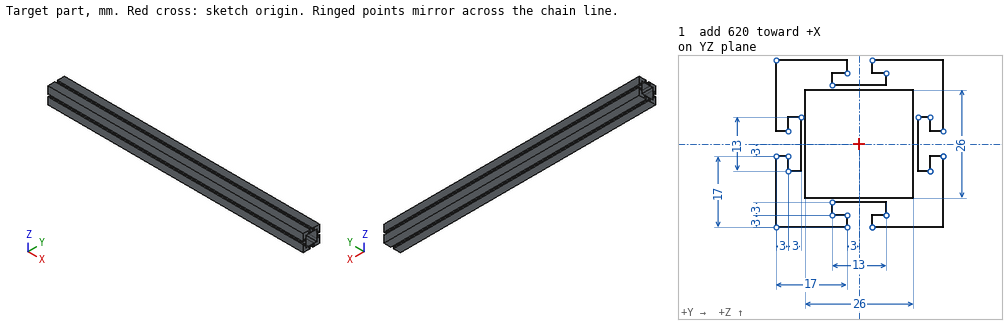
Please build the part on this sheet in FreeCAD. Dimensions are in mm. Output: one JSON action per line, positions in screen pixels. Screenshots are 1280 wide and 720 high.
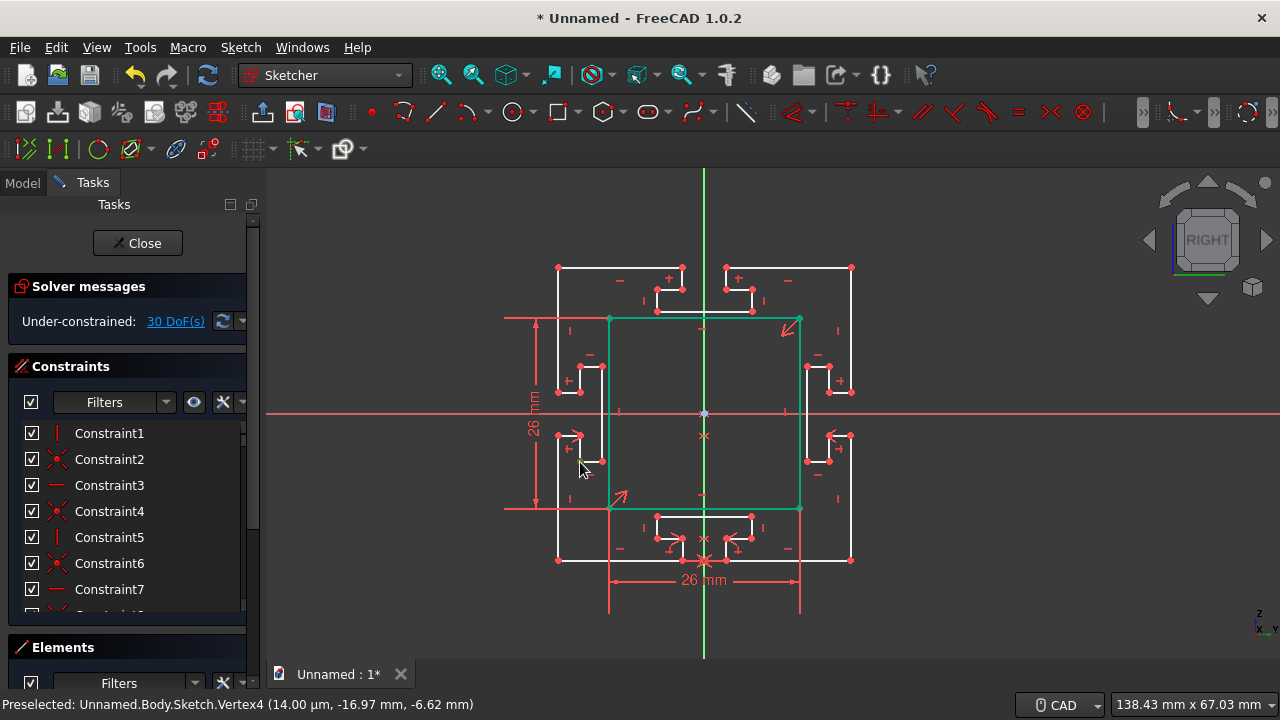
{"action": "left_click", "coordinate": [829, 462]}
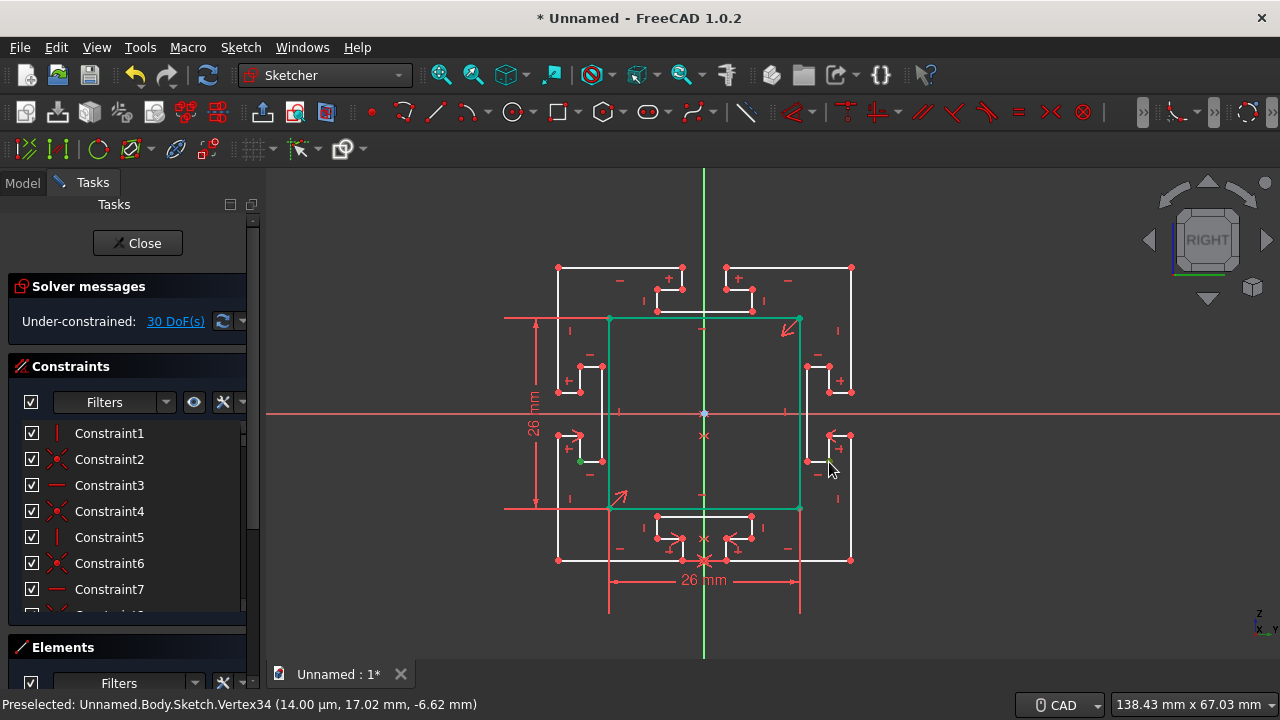
{"action": "left_click", "coordinate": [704, 600]}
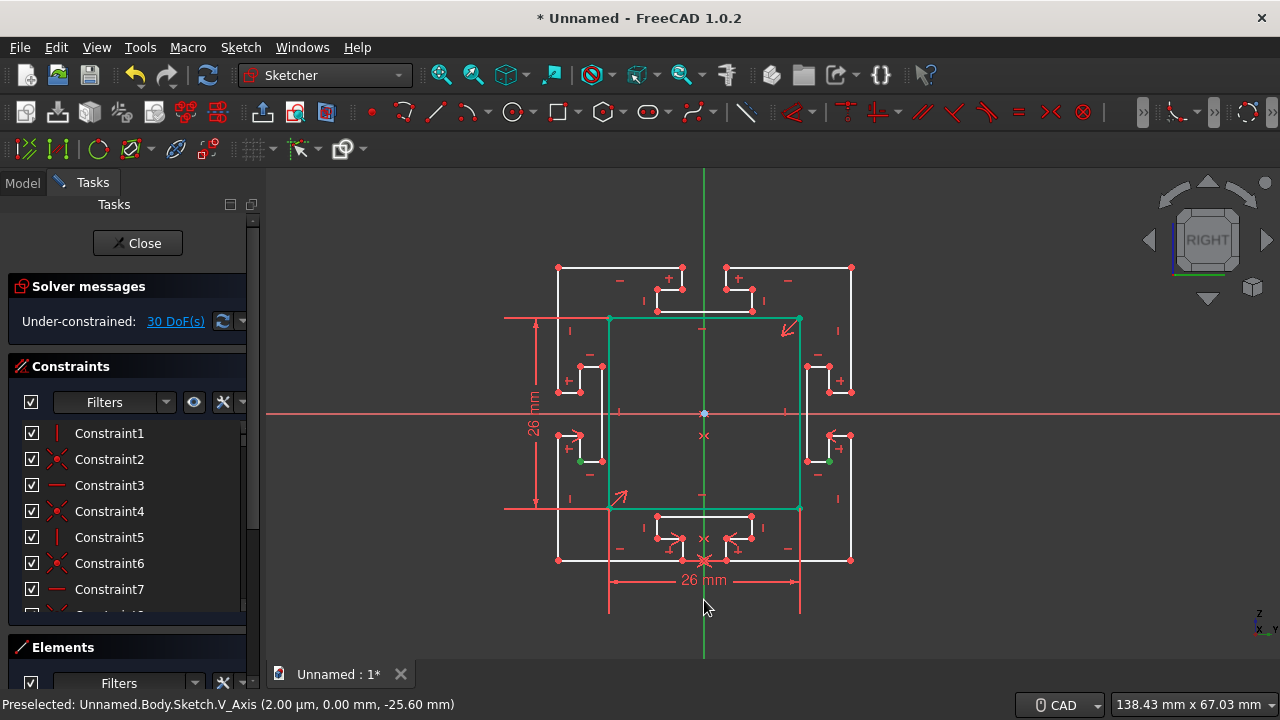
{"action": "key", "text": "s"}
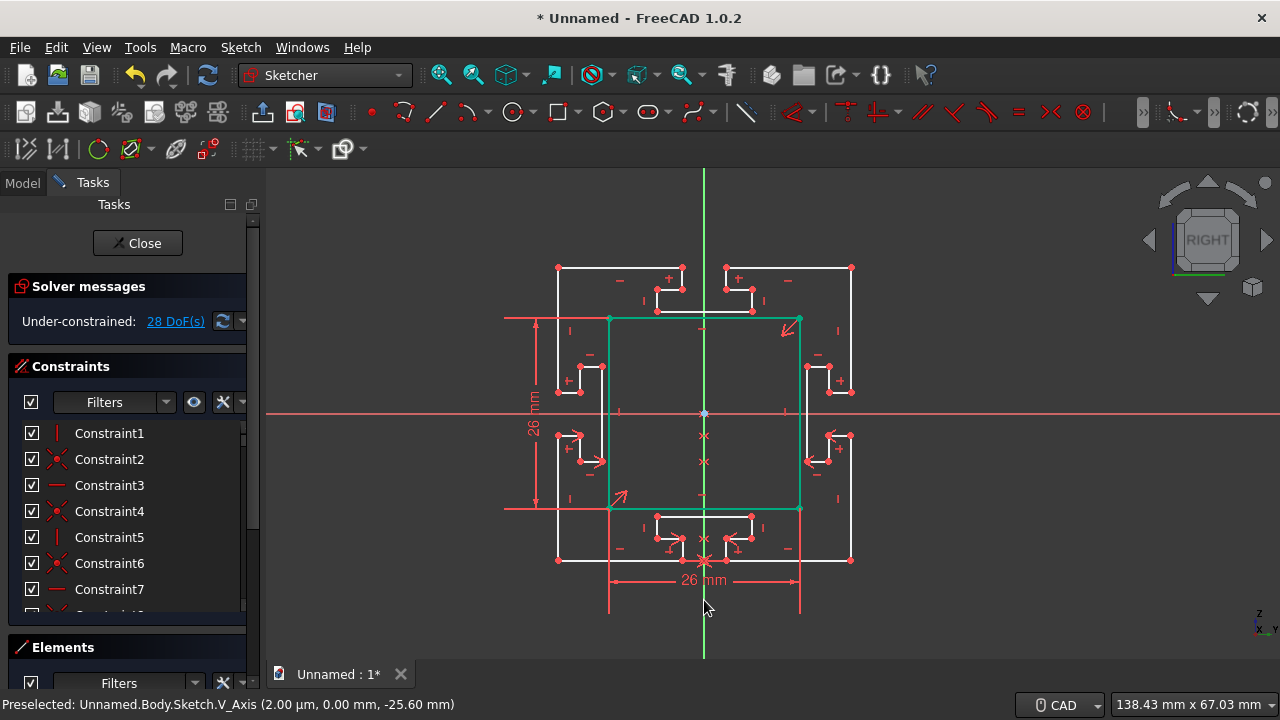
{"action": "left_click", "coordinate": [602, 367]}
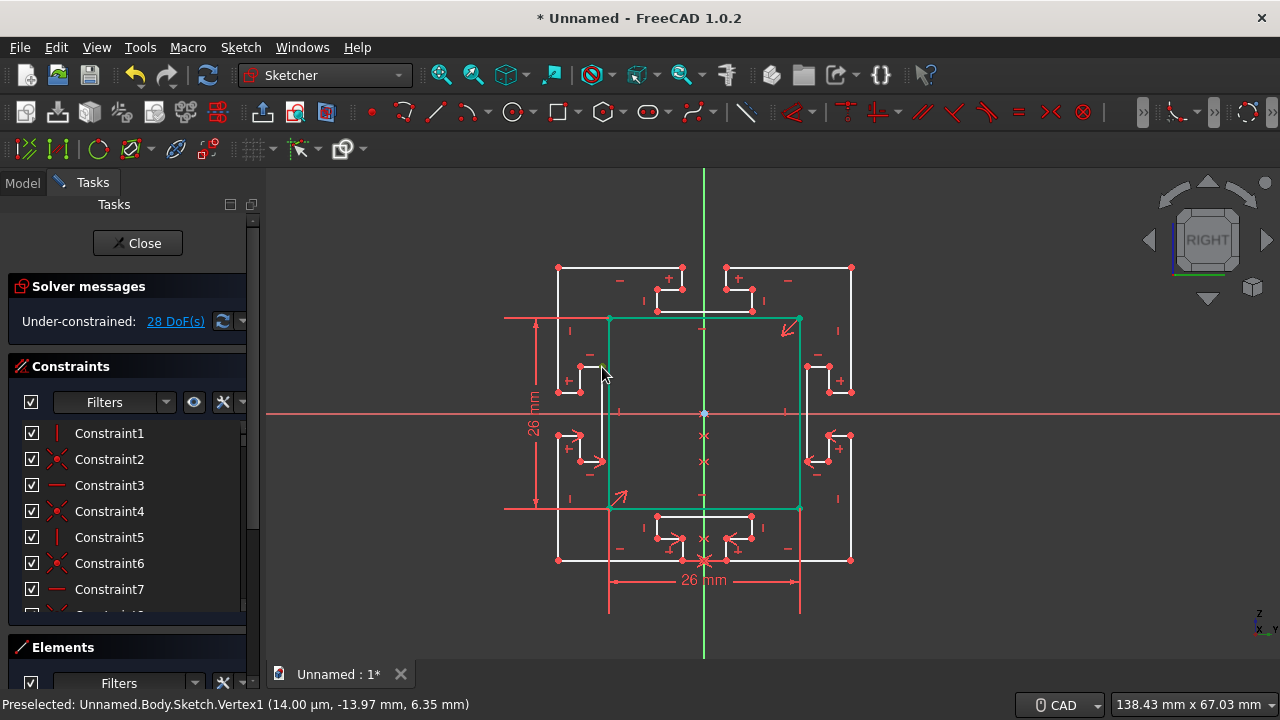
{"action": "left_click", "coordinate": [807, 367]}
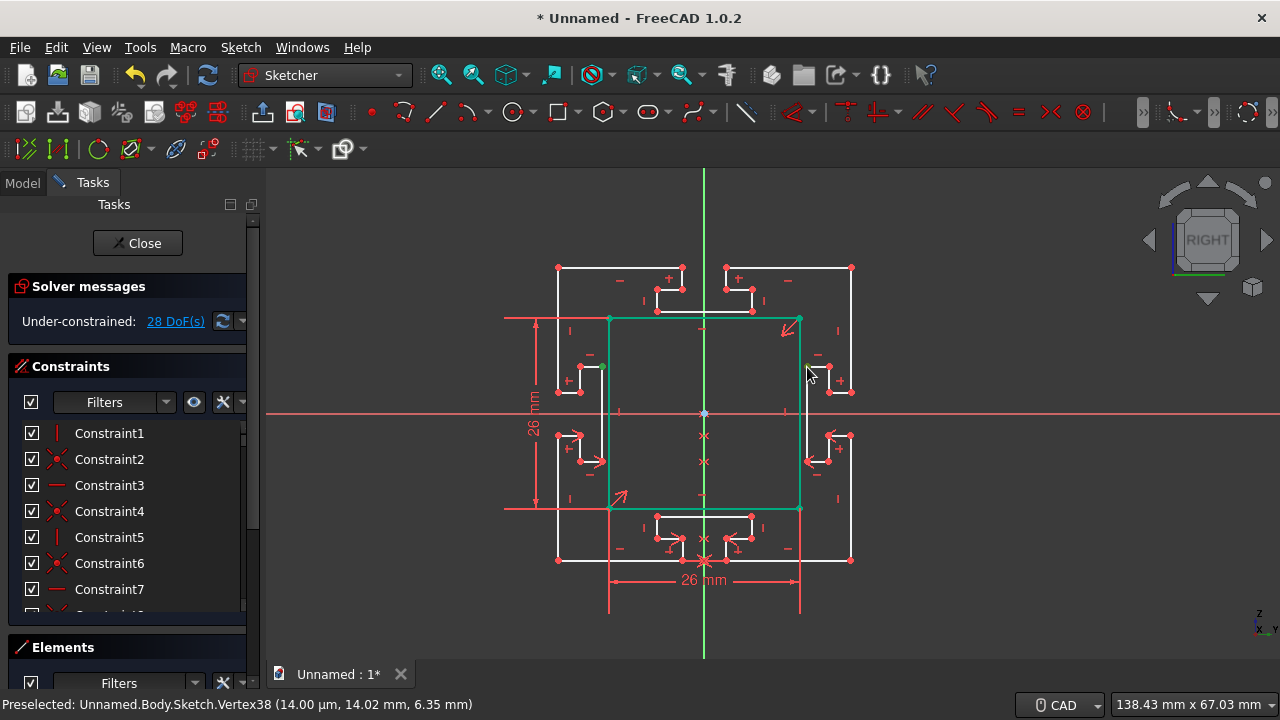
{"action": "left_click", "coordinate": [704, 600]}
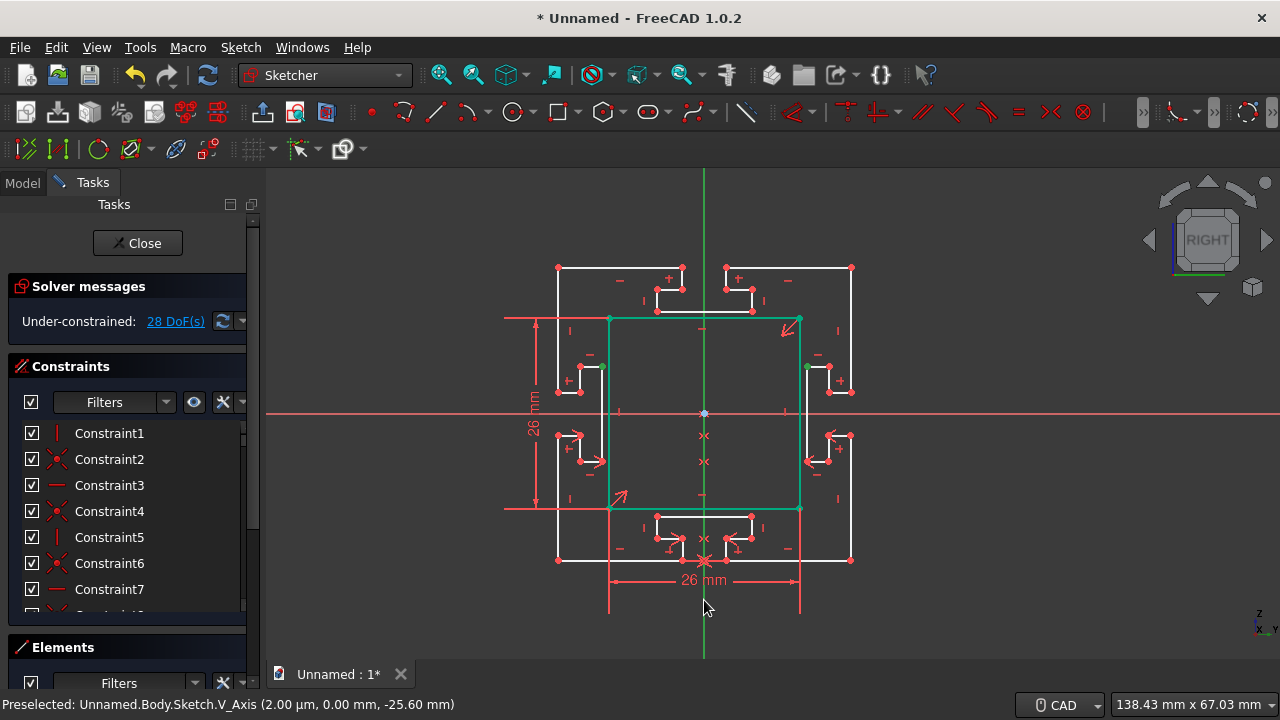
{"action": "key", "text": "s"}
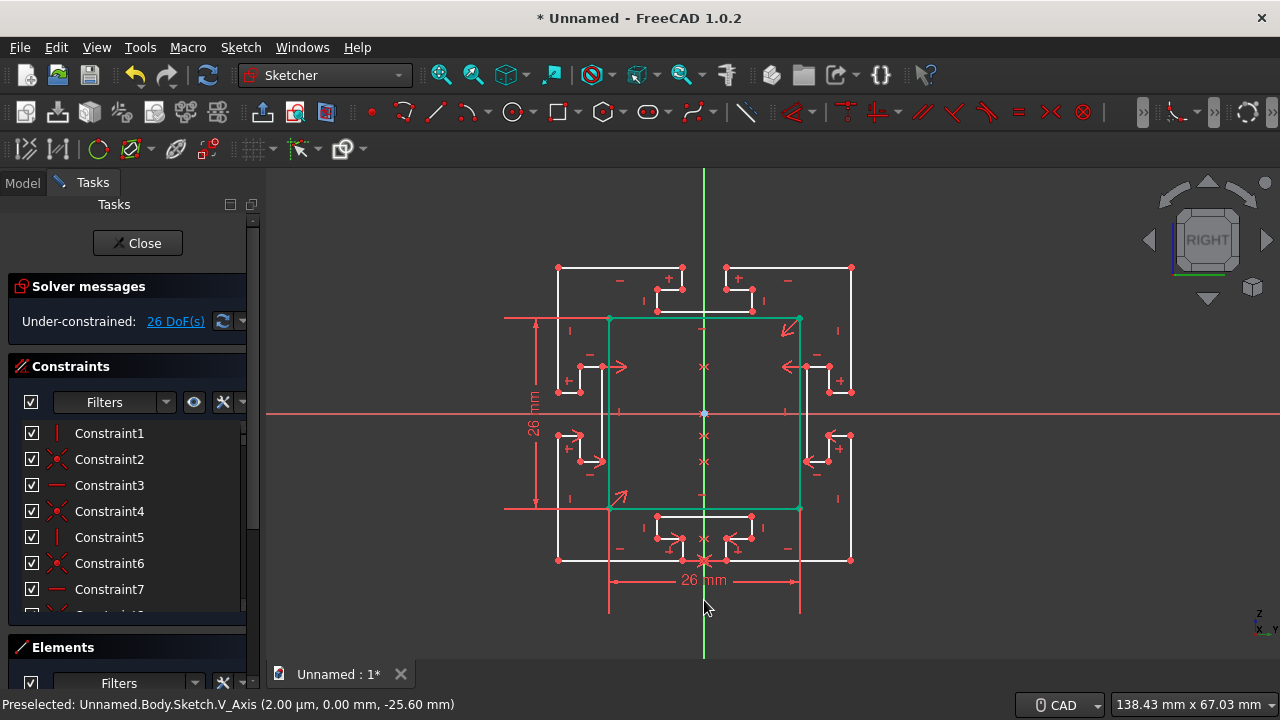
{"action": "left_click", "coordinate": [829, 462]}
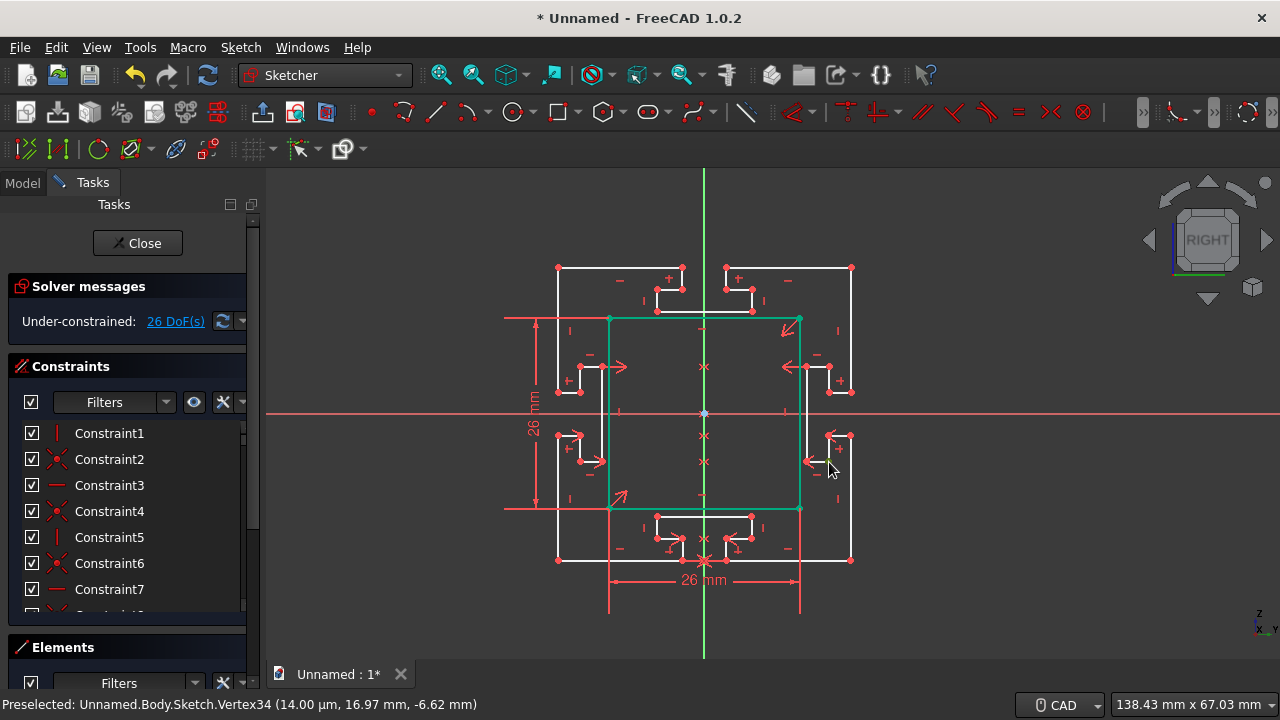
{"action": "left_click", "coordinate": [829, 367]}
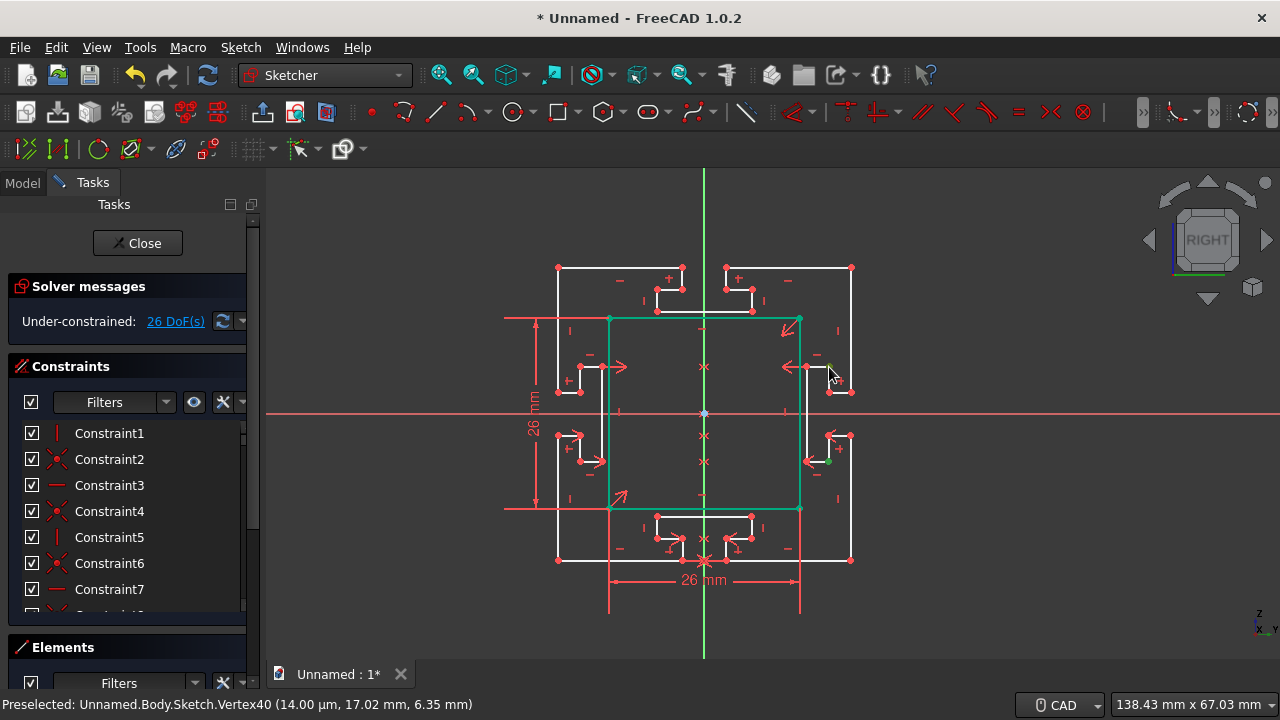
{"action": "left_click", "coordinate": [353, 414]}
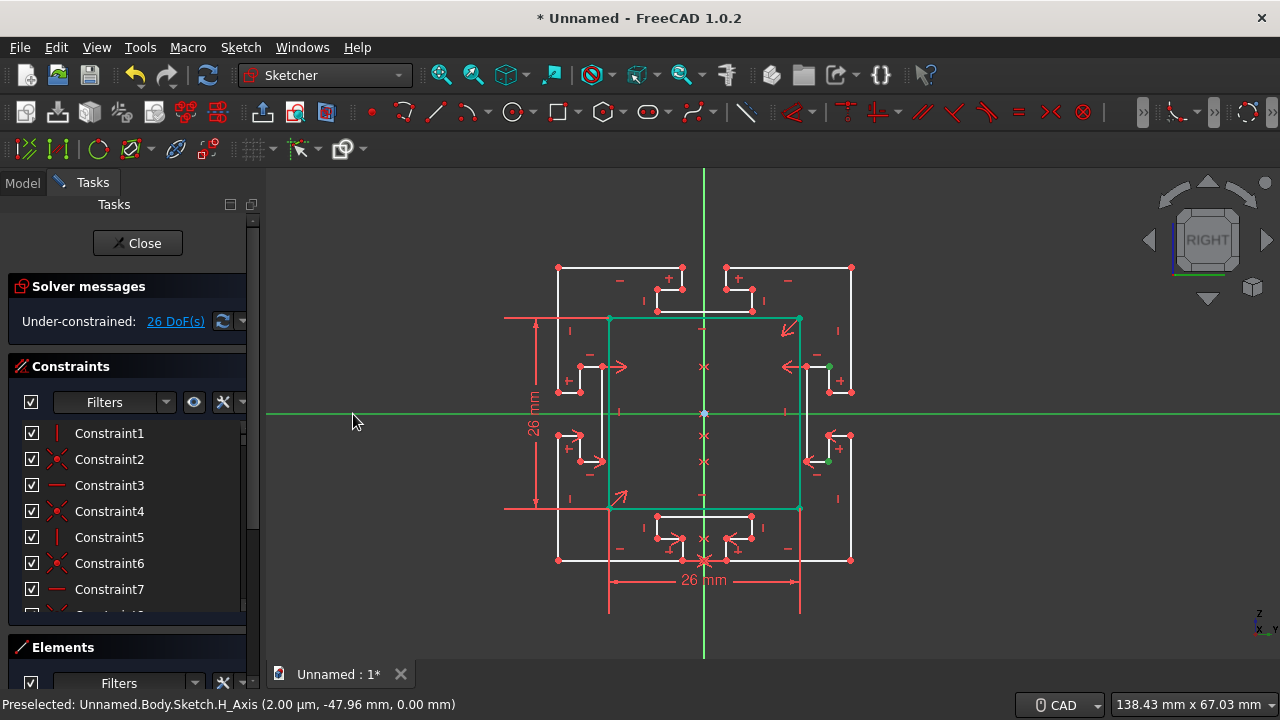
{"action": "key", "text": "s"}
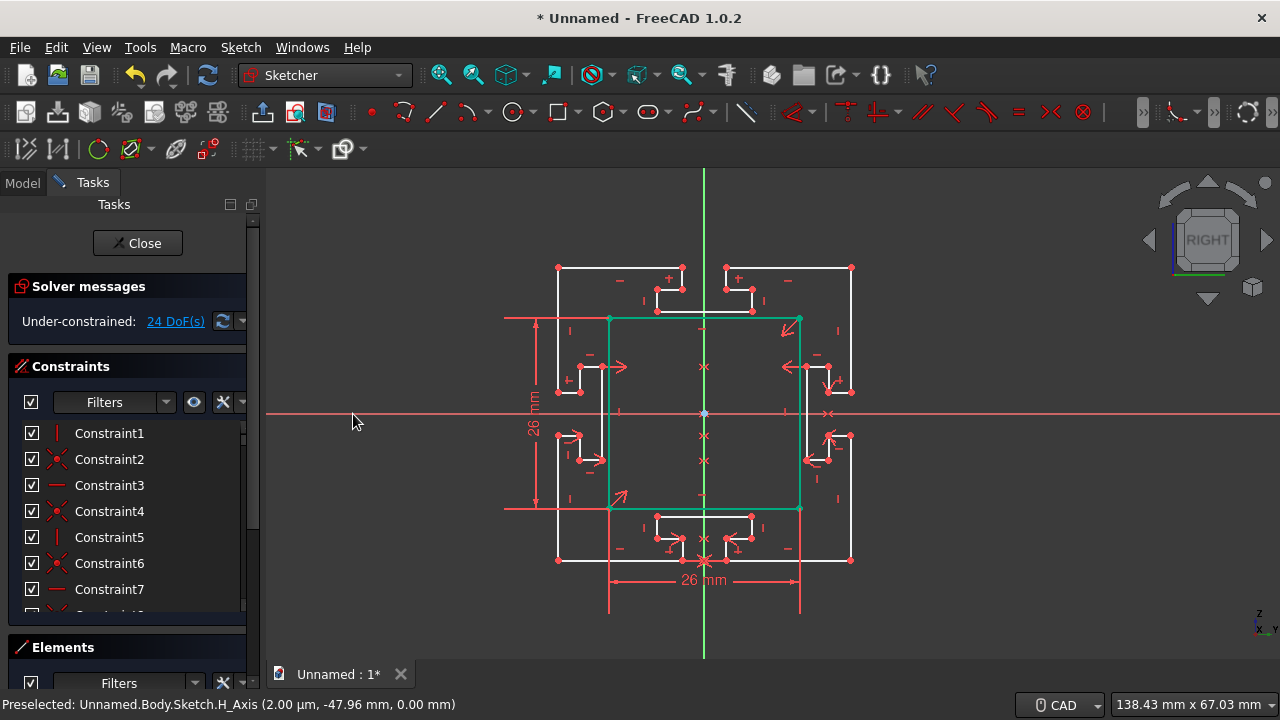
{"action": "left_click", "coordinate": [851, 436]}